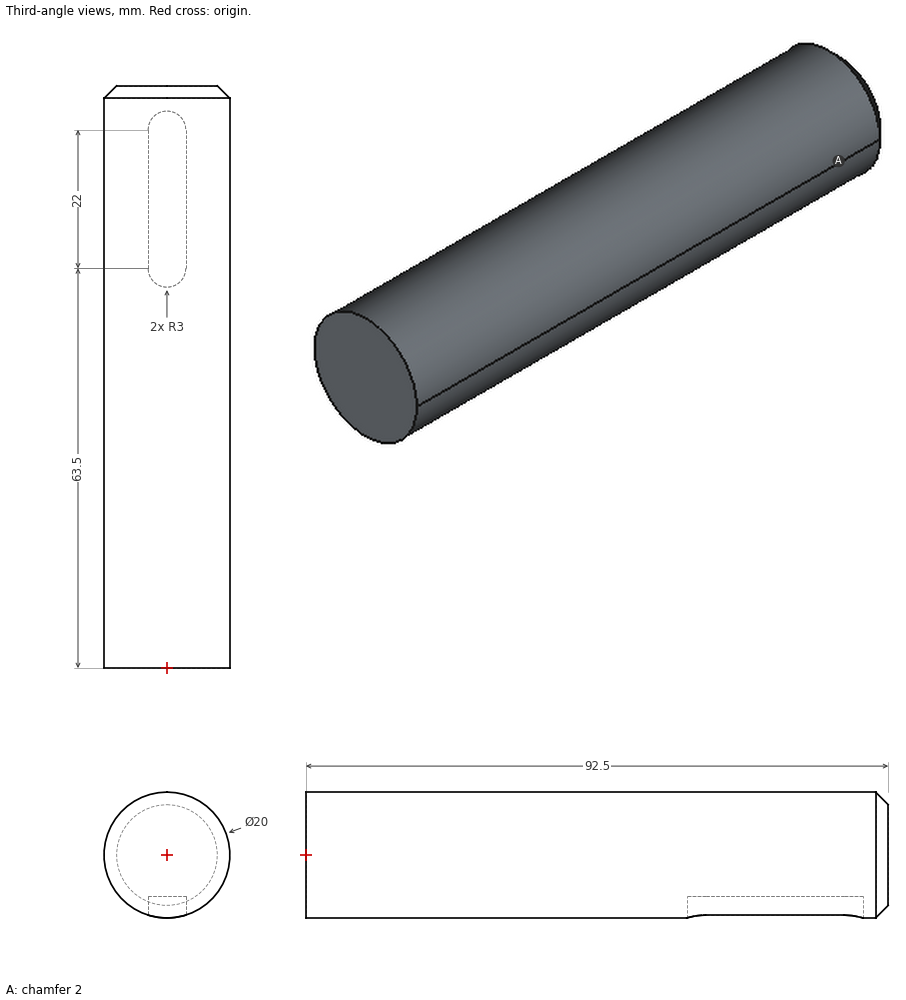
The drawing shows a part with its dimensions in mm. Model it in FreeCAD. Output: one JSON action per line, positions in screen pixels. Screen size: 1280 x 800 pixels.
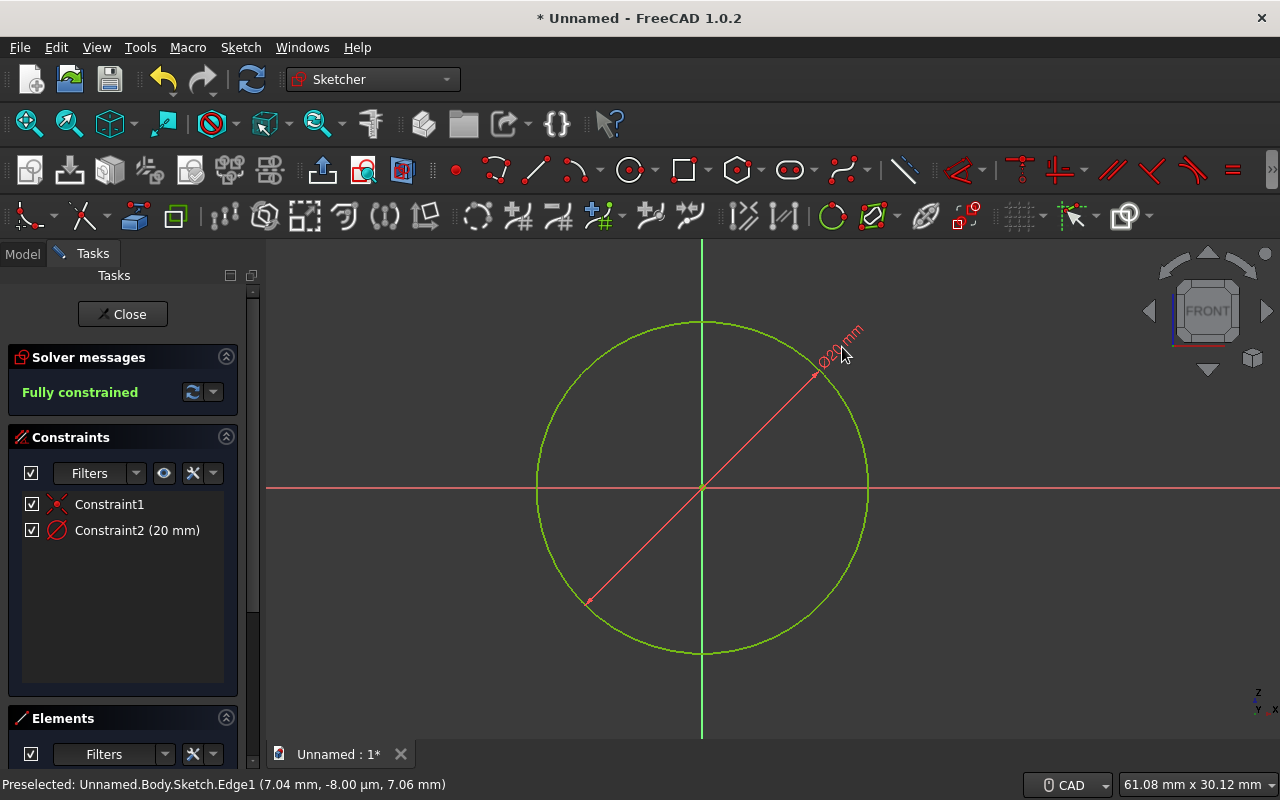
{"action": "left_click", "coordinate": [123, 314]}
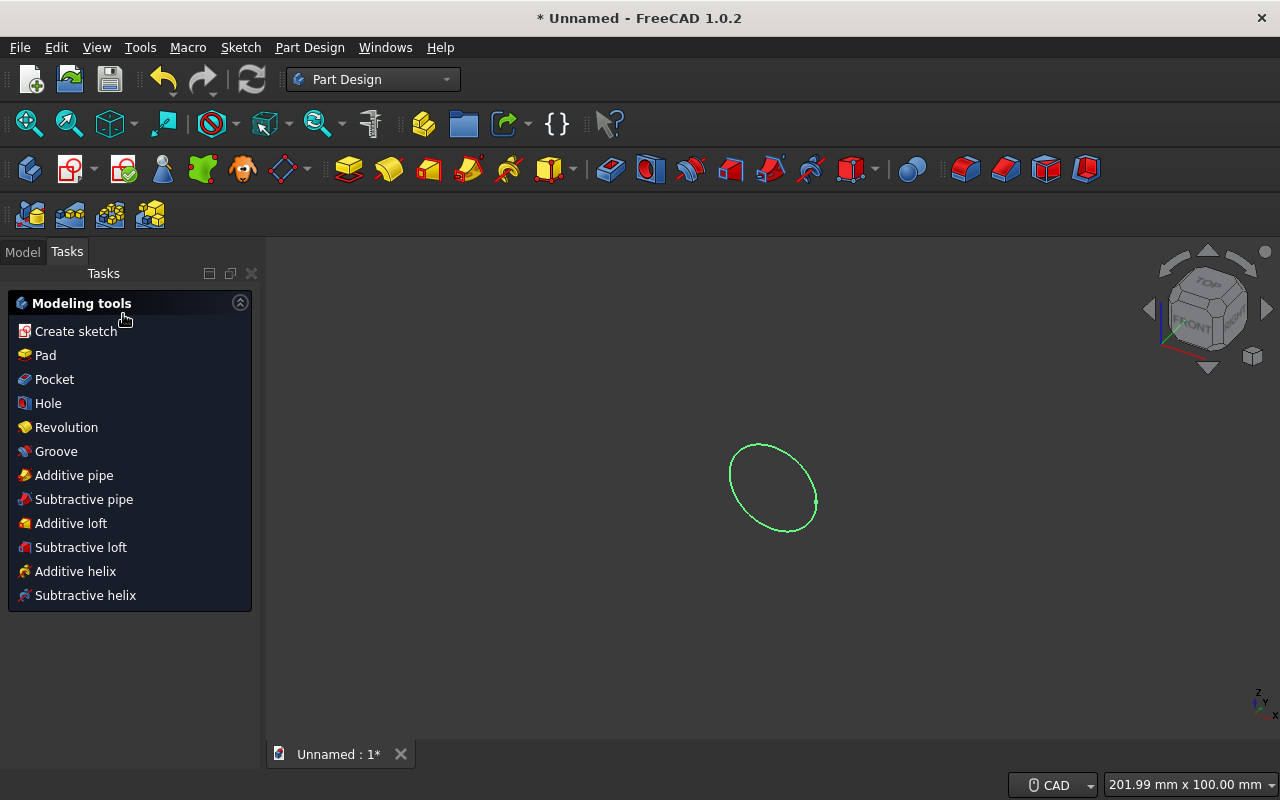
{"action": "left_click", "coordinate": [350, 170]}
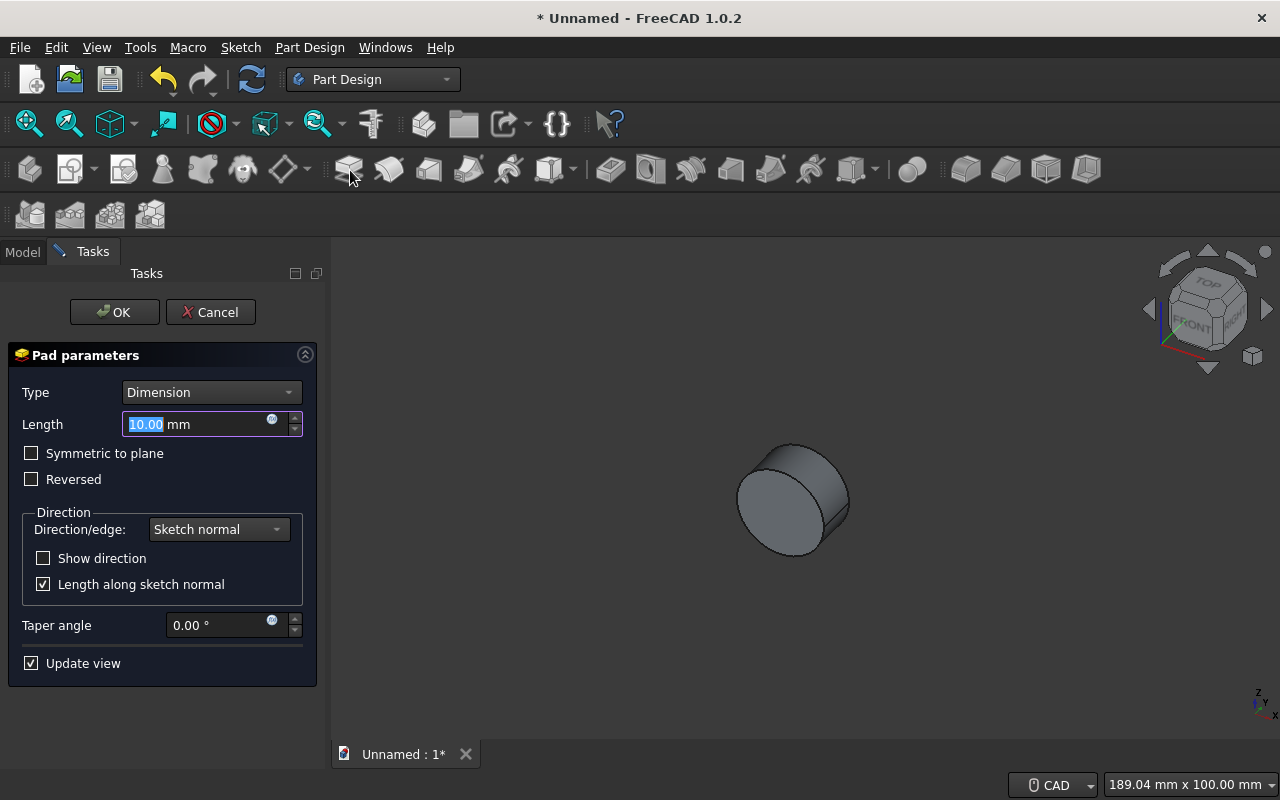
{"action": "type", "text": "92.5"}
{"action": "key", "text": "Tab"}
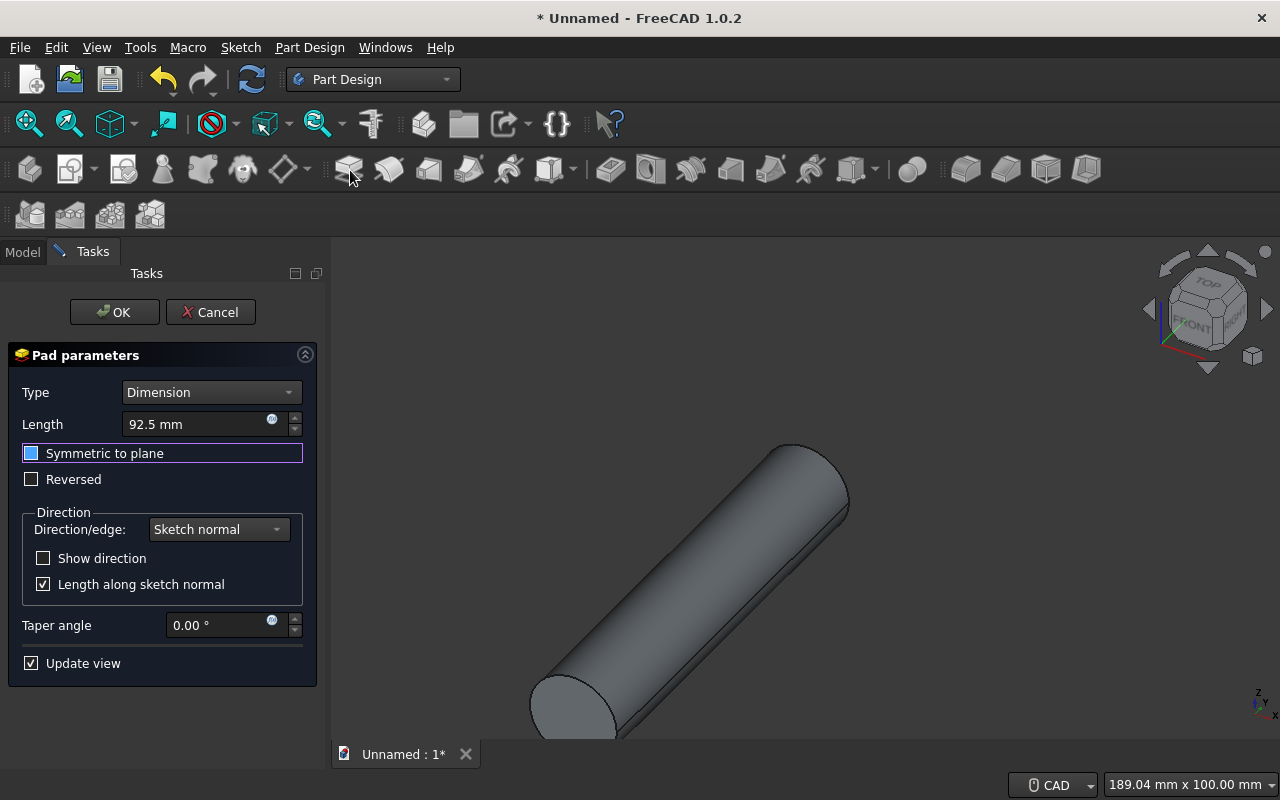
{"action": "left_click", "coordinate": [30, 479]}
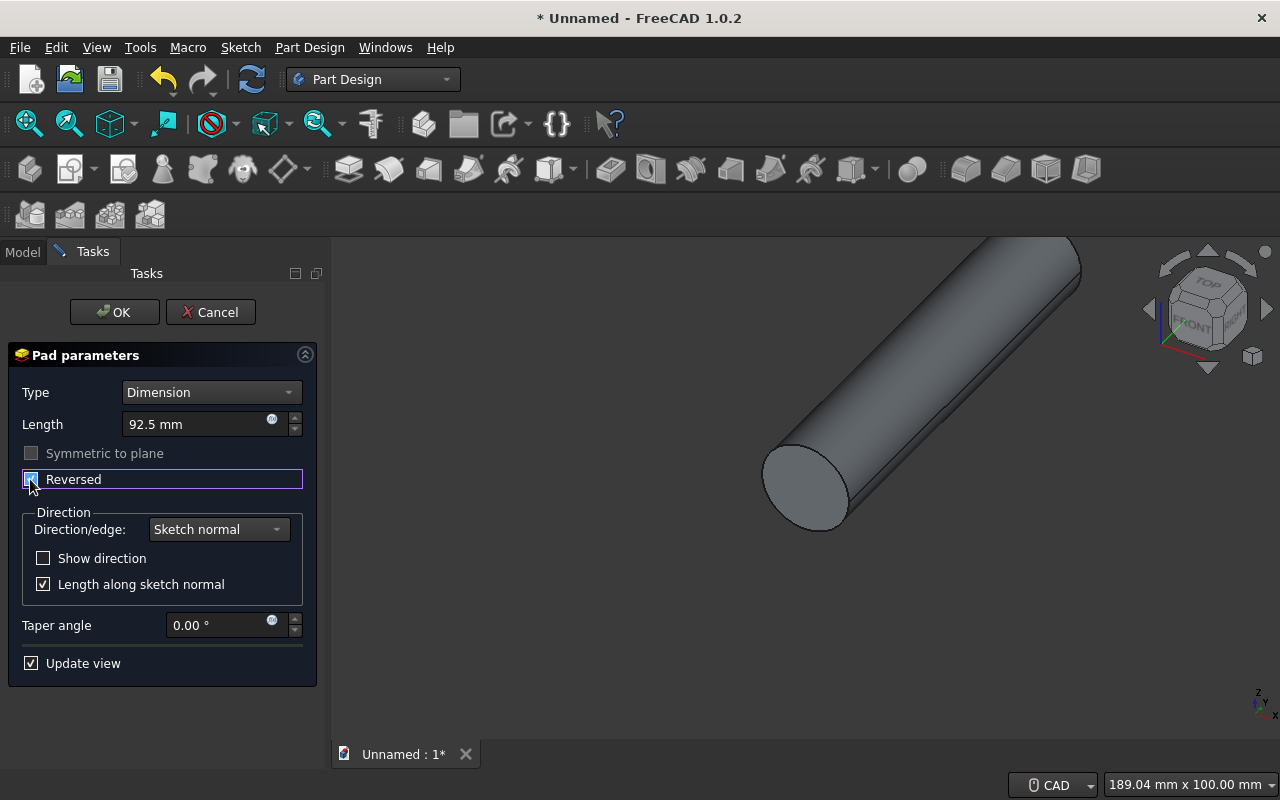
{"action": "left_click", "coordinate": [115, 312]}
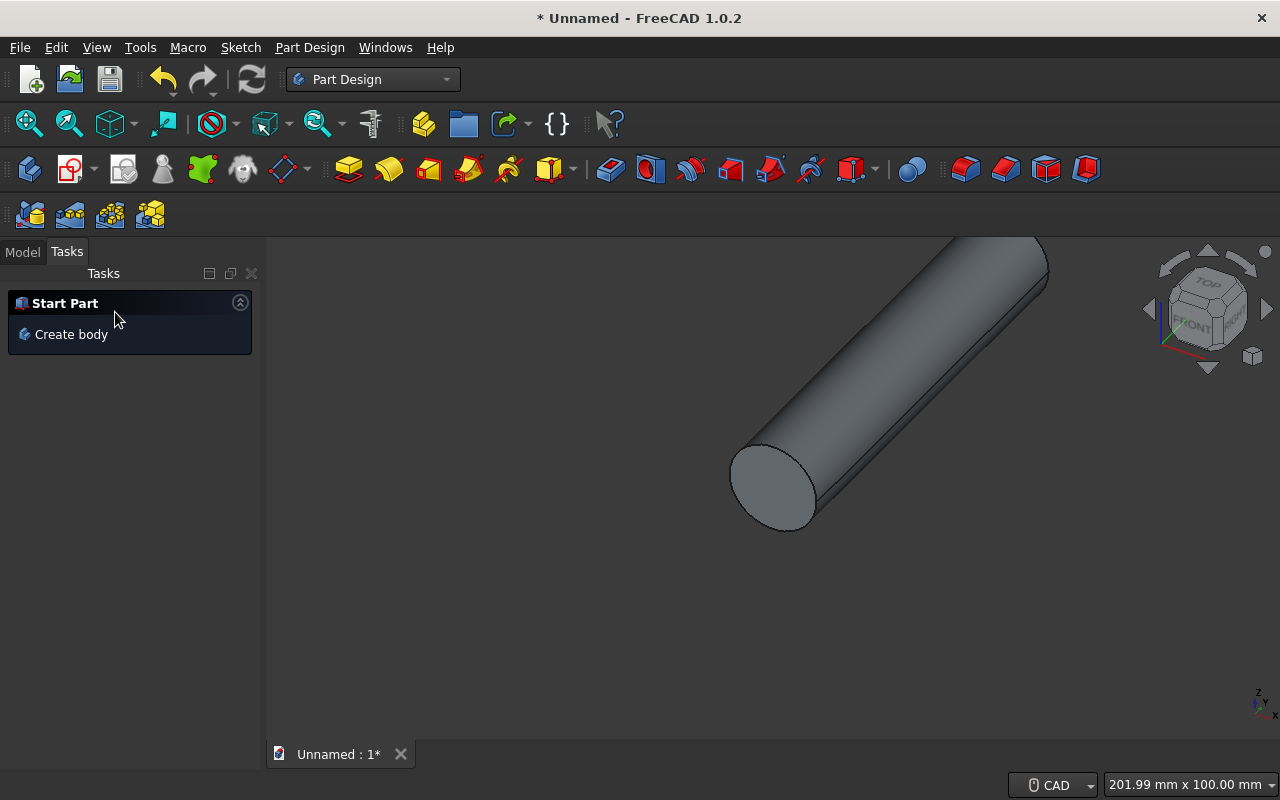
{"action": "left_click", "coordinate": [30, 124]}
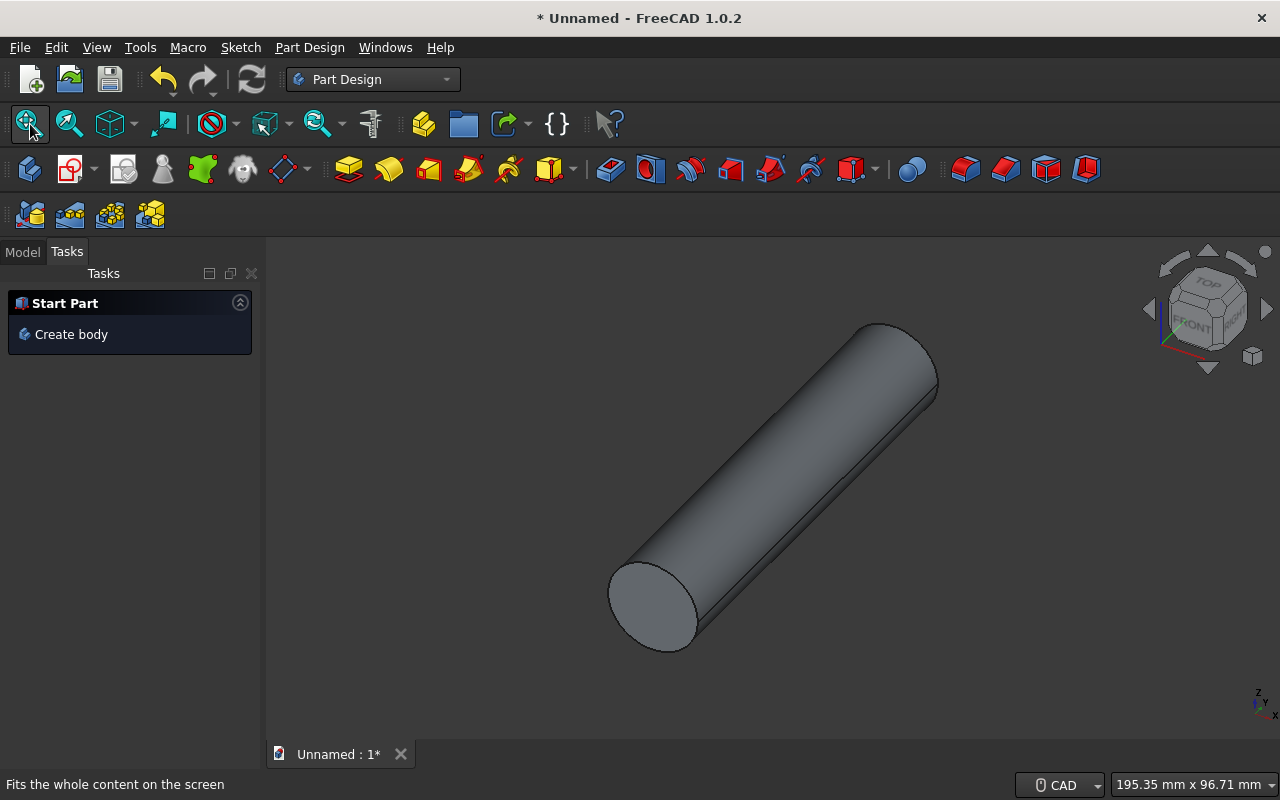
{"action": "left_click", "coordinate": [23, 251]}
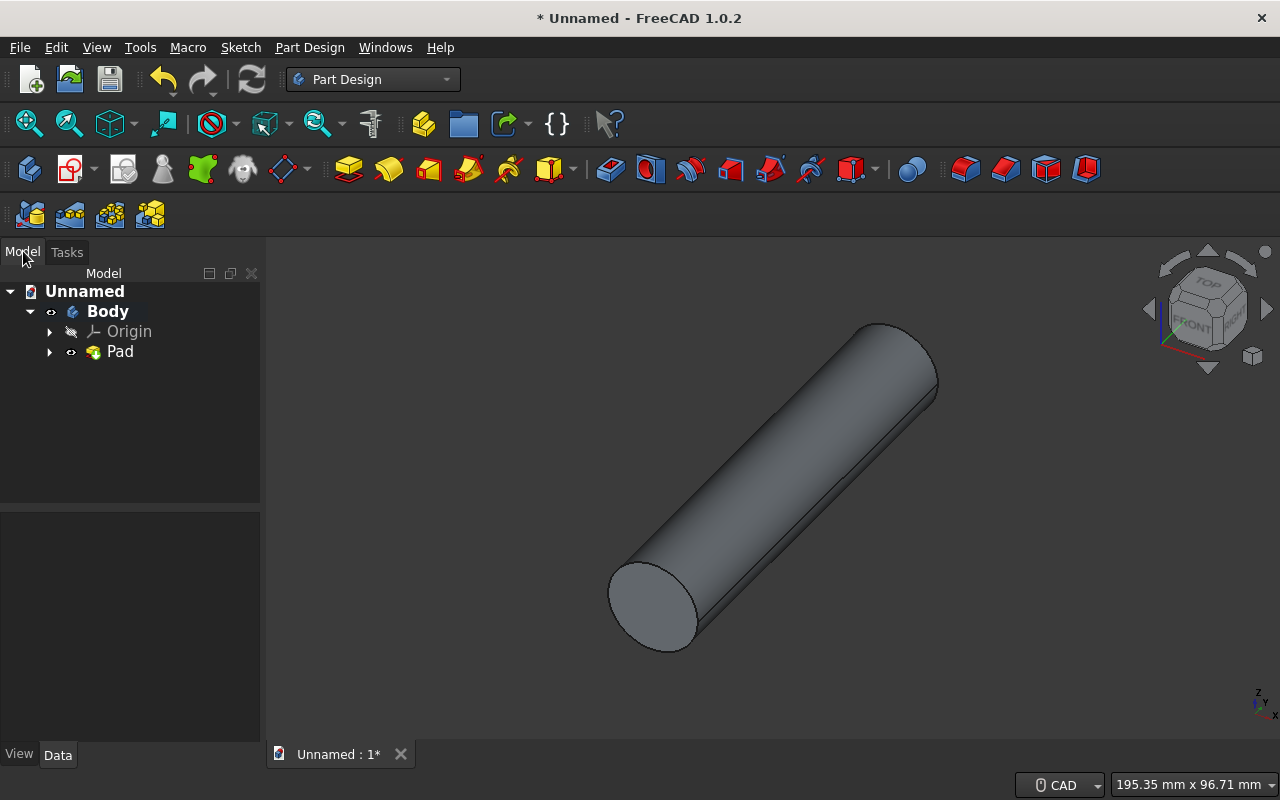
{"action": "left_click", "coordinate": [50, 332]}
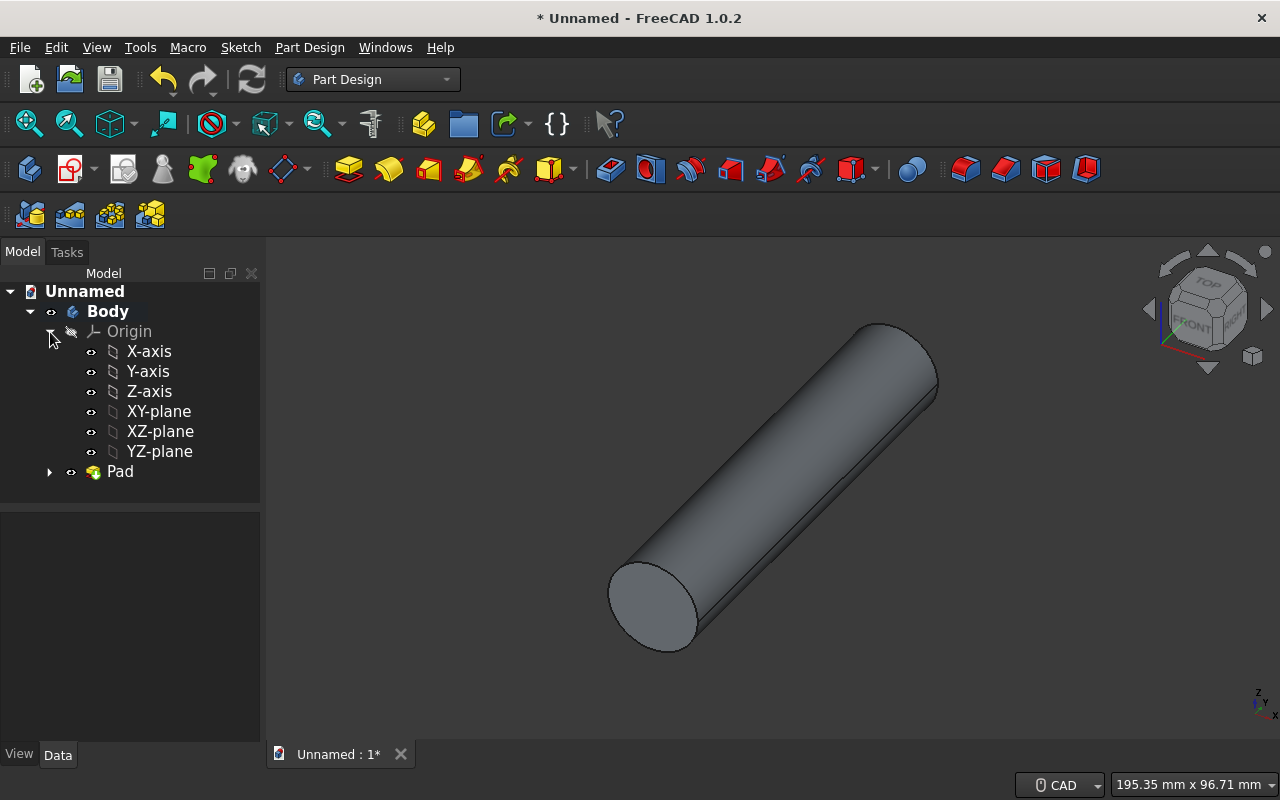
{"action": "left_click", "coordinate": [136, 412]}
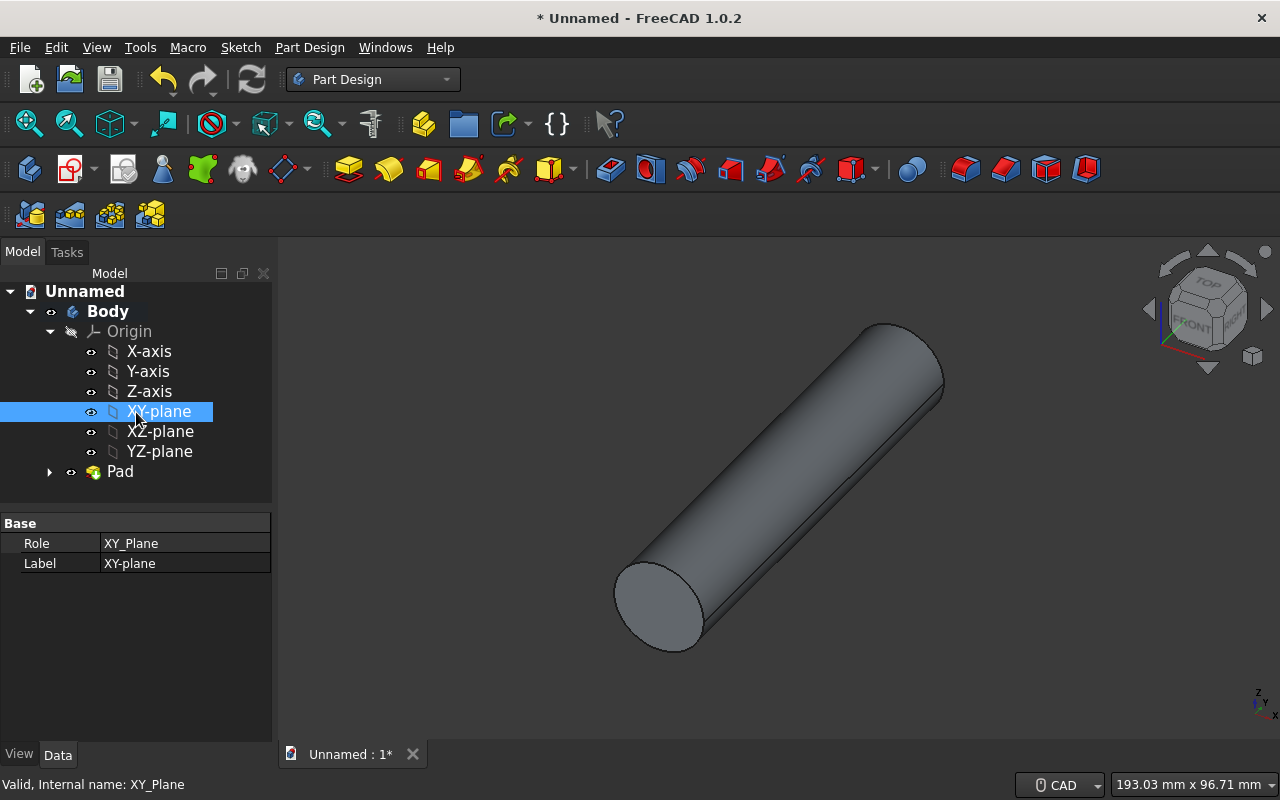
{"action": "left_click", "coordinate": [284, 170]}